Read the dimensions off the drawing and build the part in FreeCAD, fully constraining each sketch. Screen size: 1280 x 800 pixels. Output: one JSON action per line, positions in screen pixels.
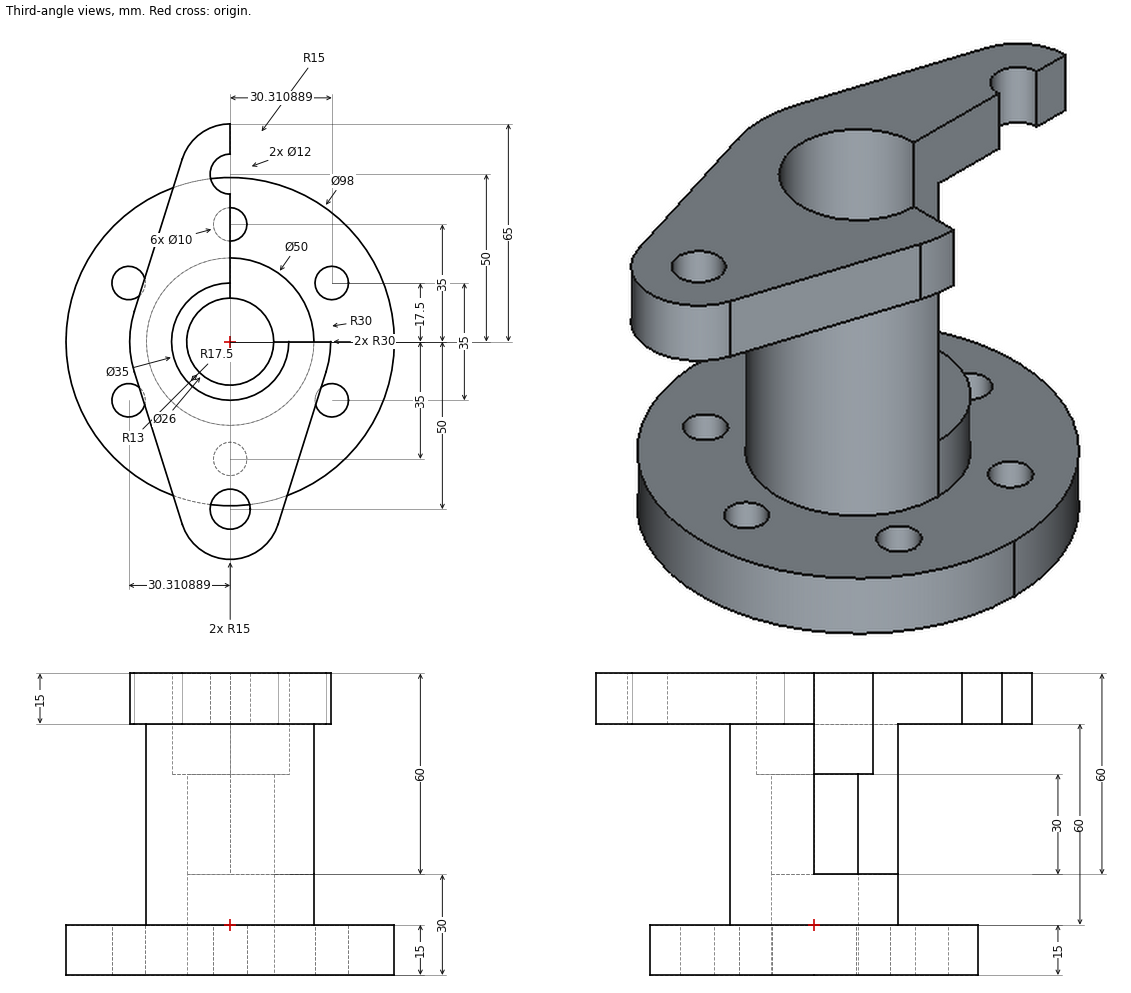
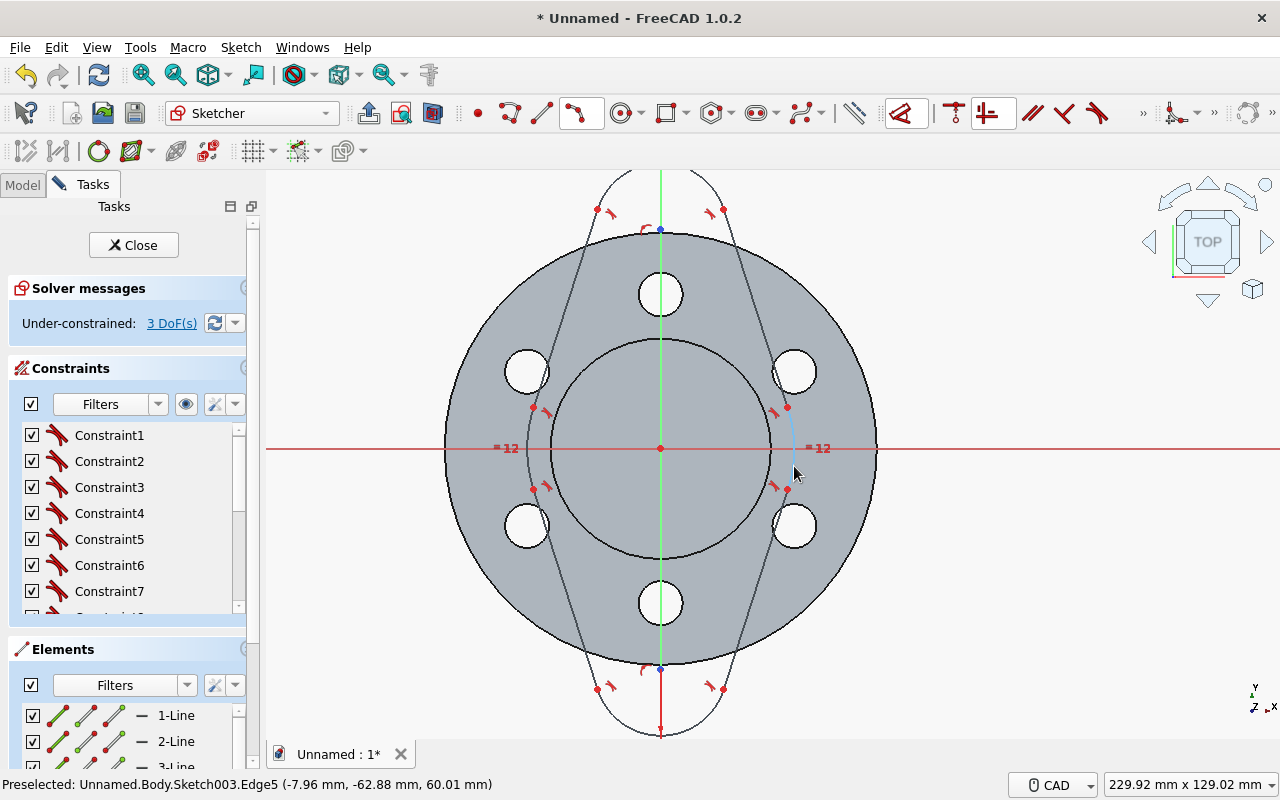
{"action": "left_click", "coordinate": [793, 465]}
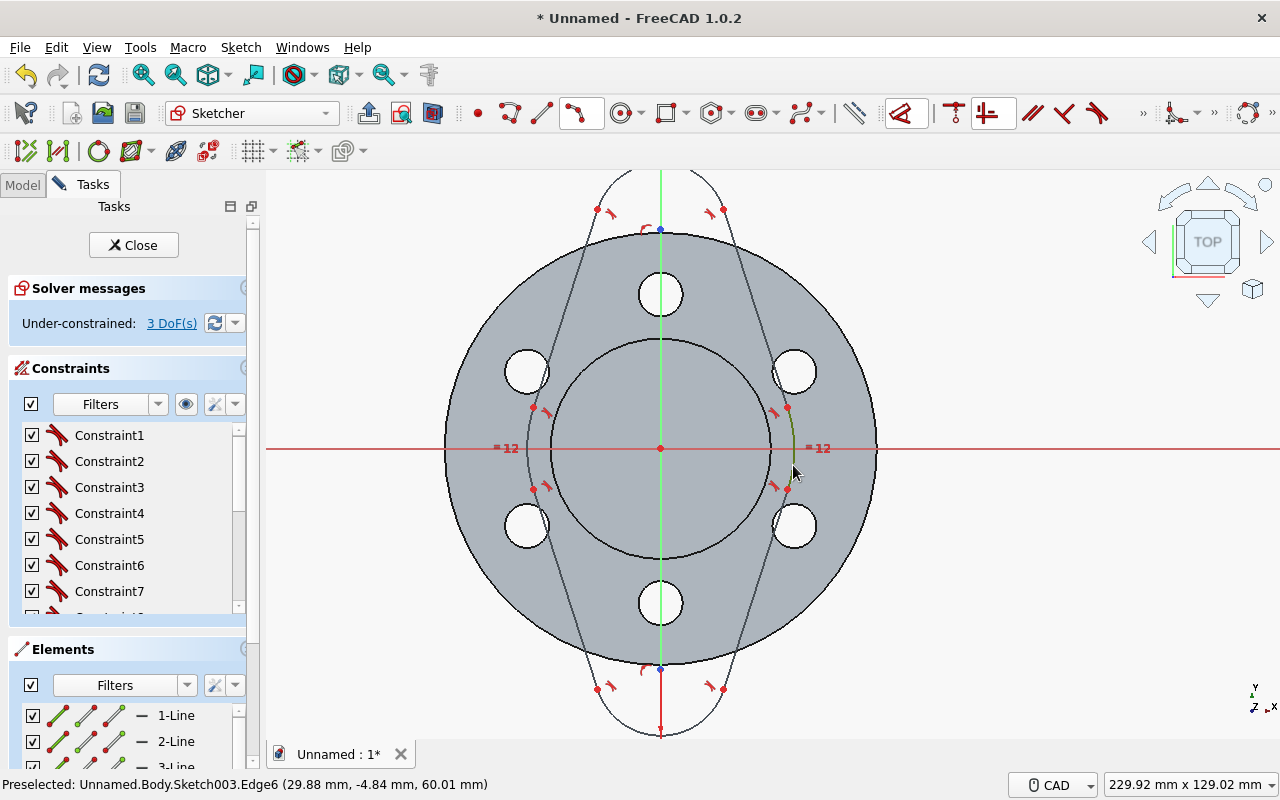
{"action": "key", "text": "k r"}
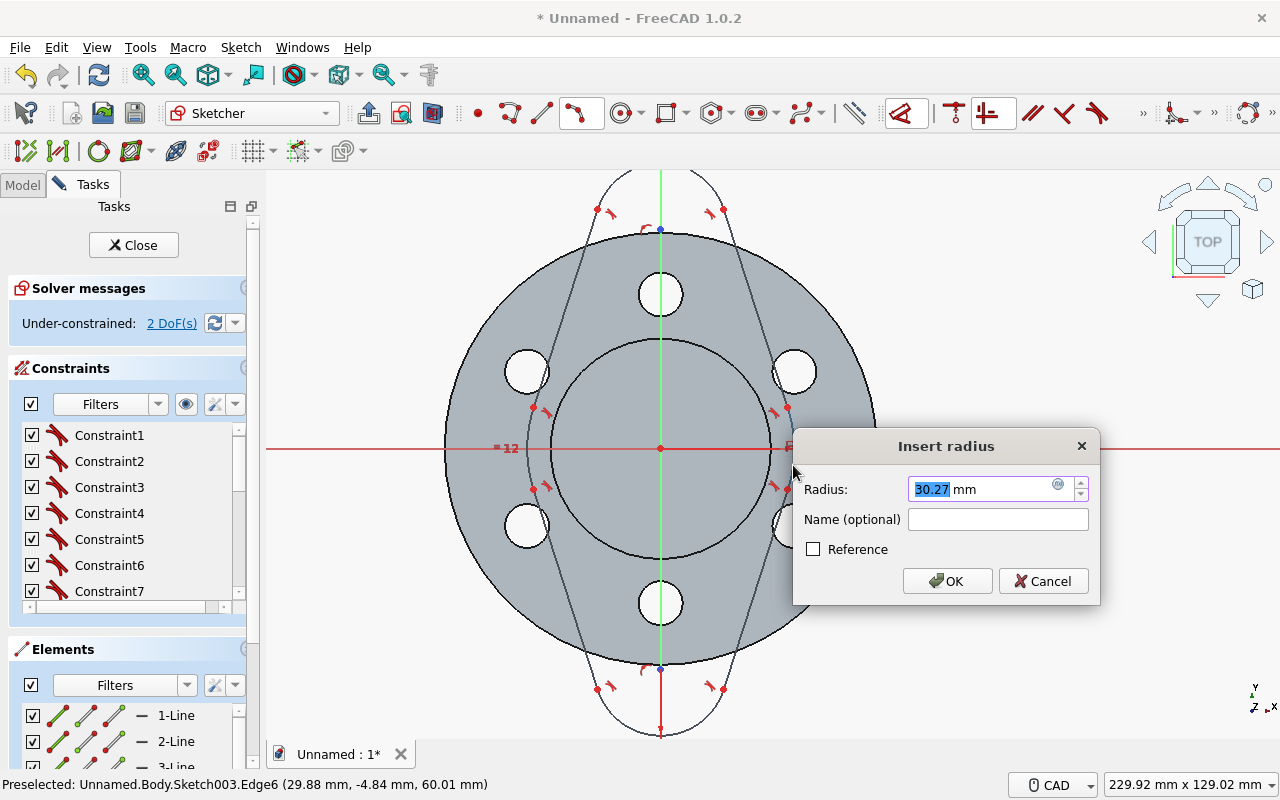
{"action": "type", "text": "30"}
{"action": "key", "text": "Return"}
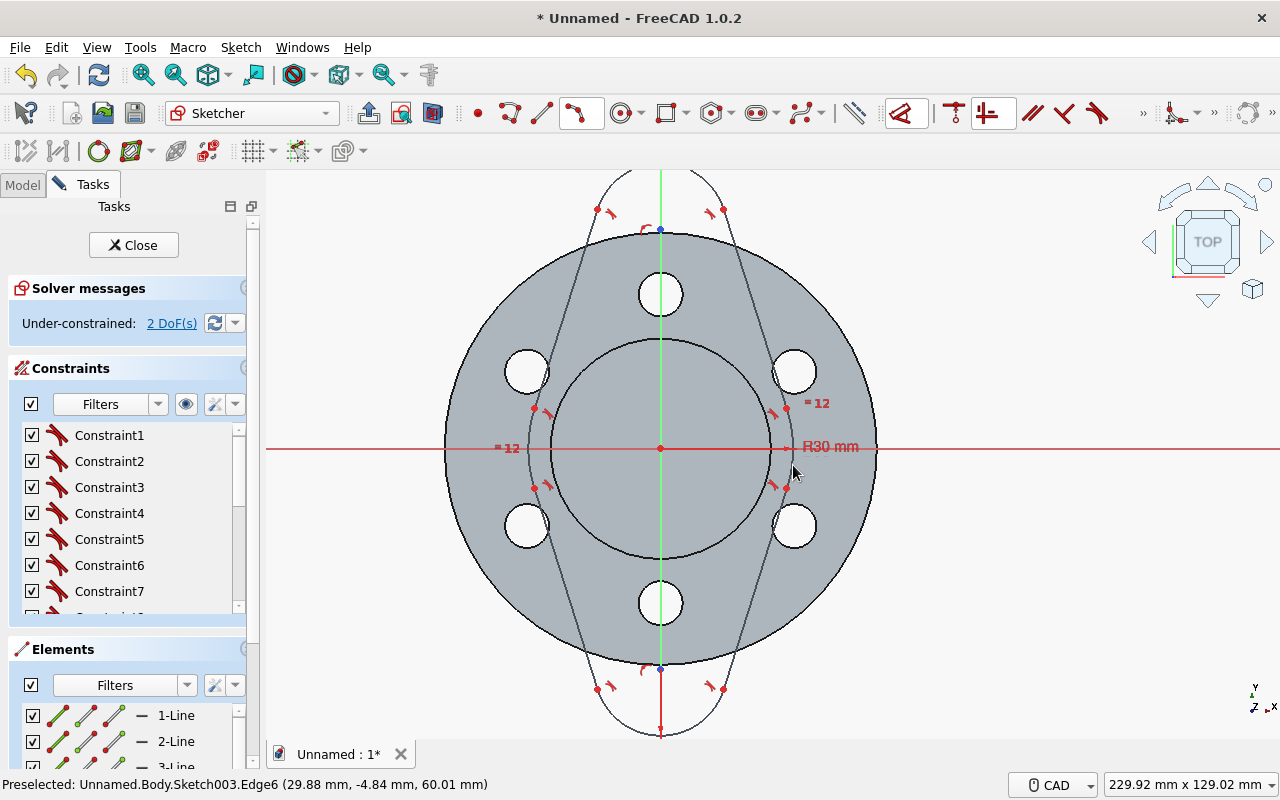
{"action": "left_click", "coordinate": [661, 670]}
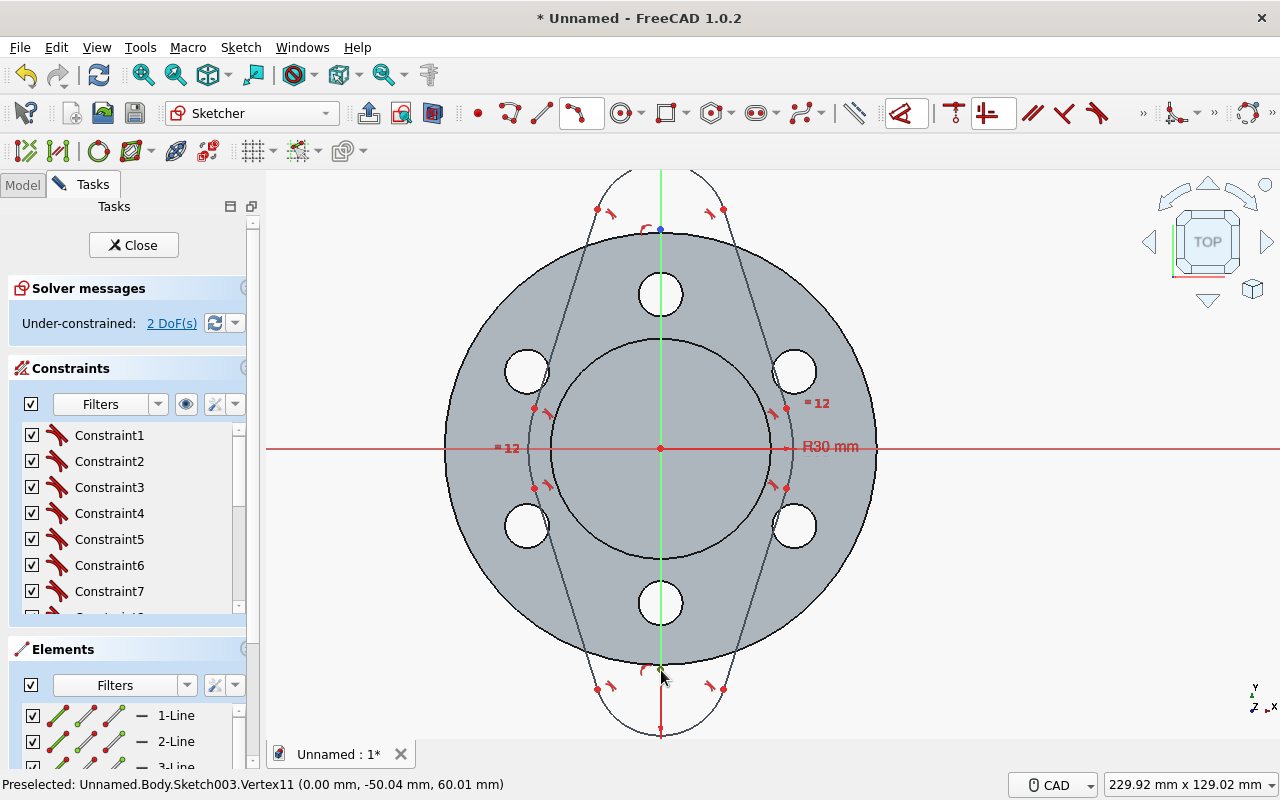
{"action": "key", "text": "i"}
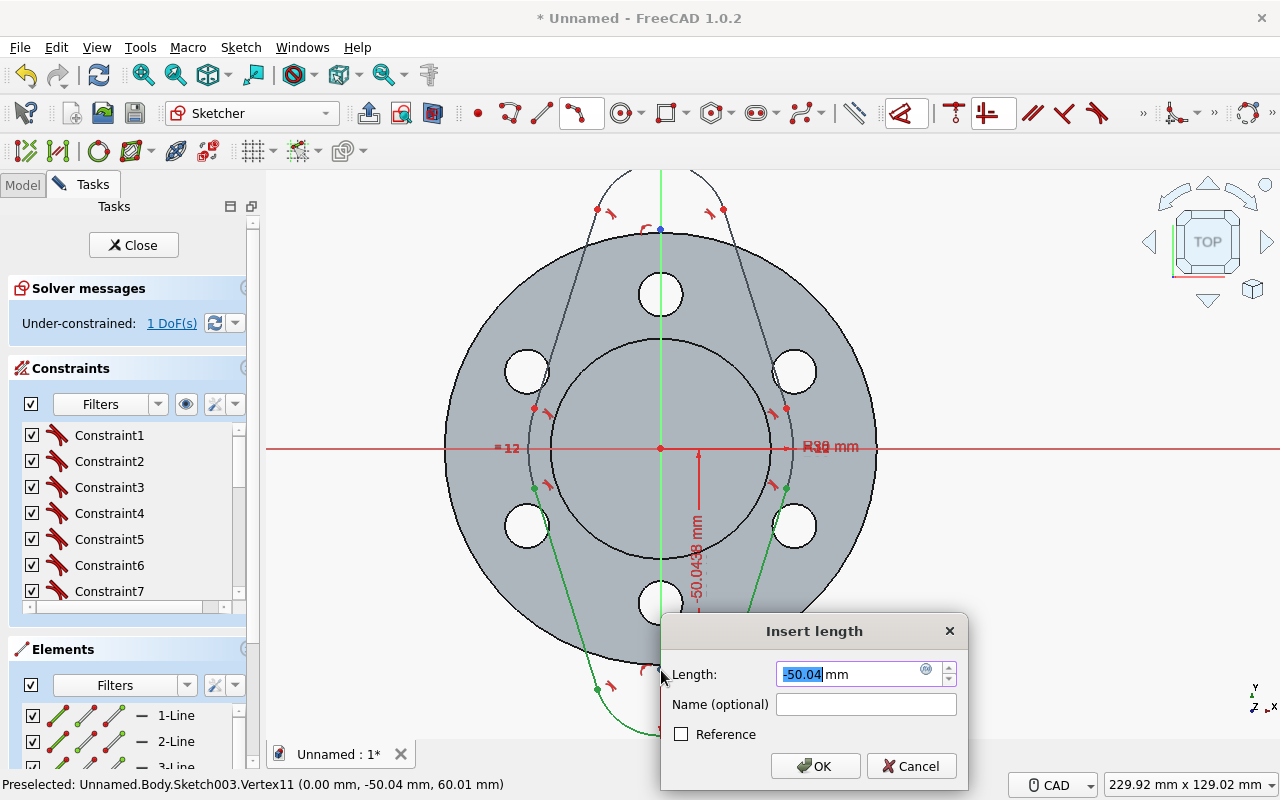
{"action": "type", "text": "-50"}
{"action": "key", "text": "Return"}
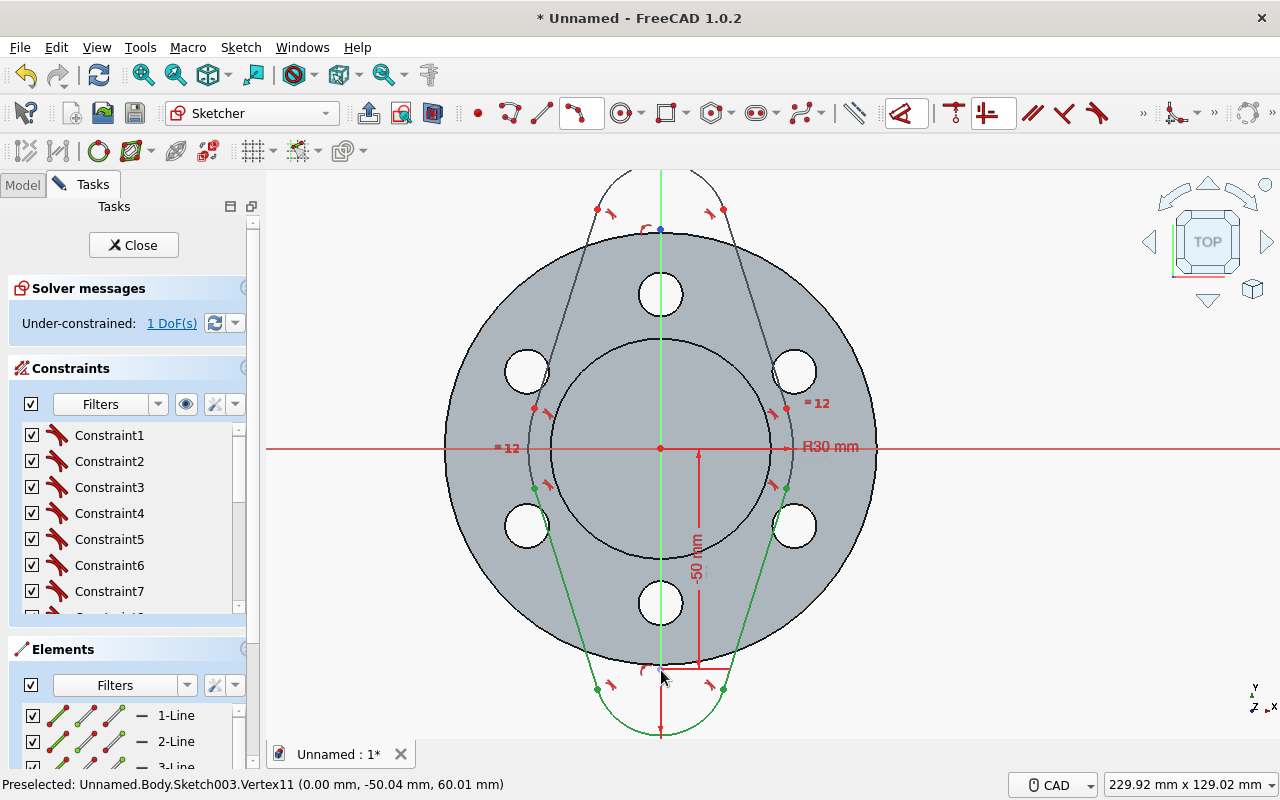
{"action": "left_click", "coordinate": [661, 230]}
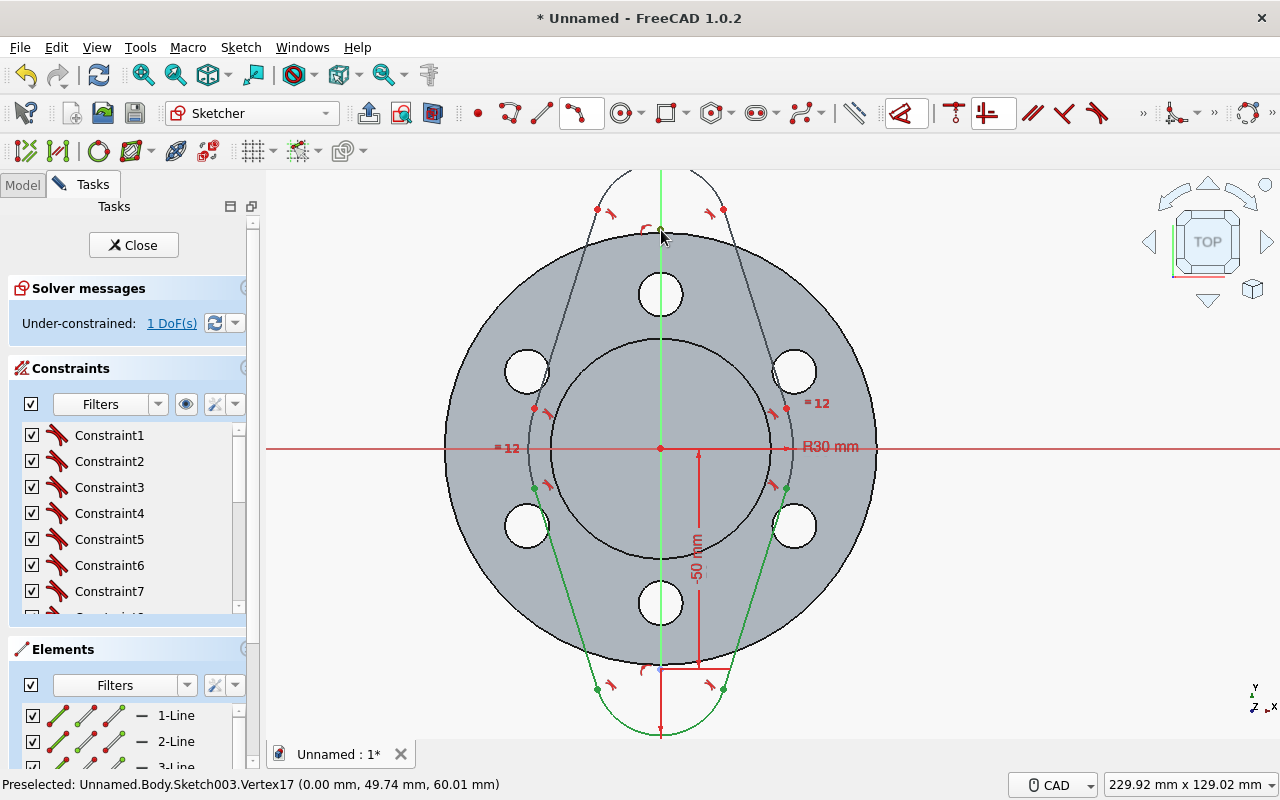
{"action": "key", "text": "i"}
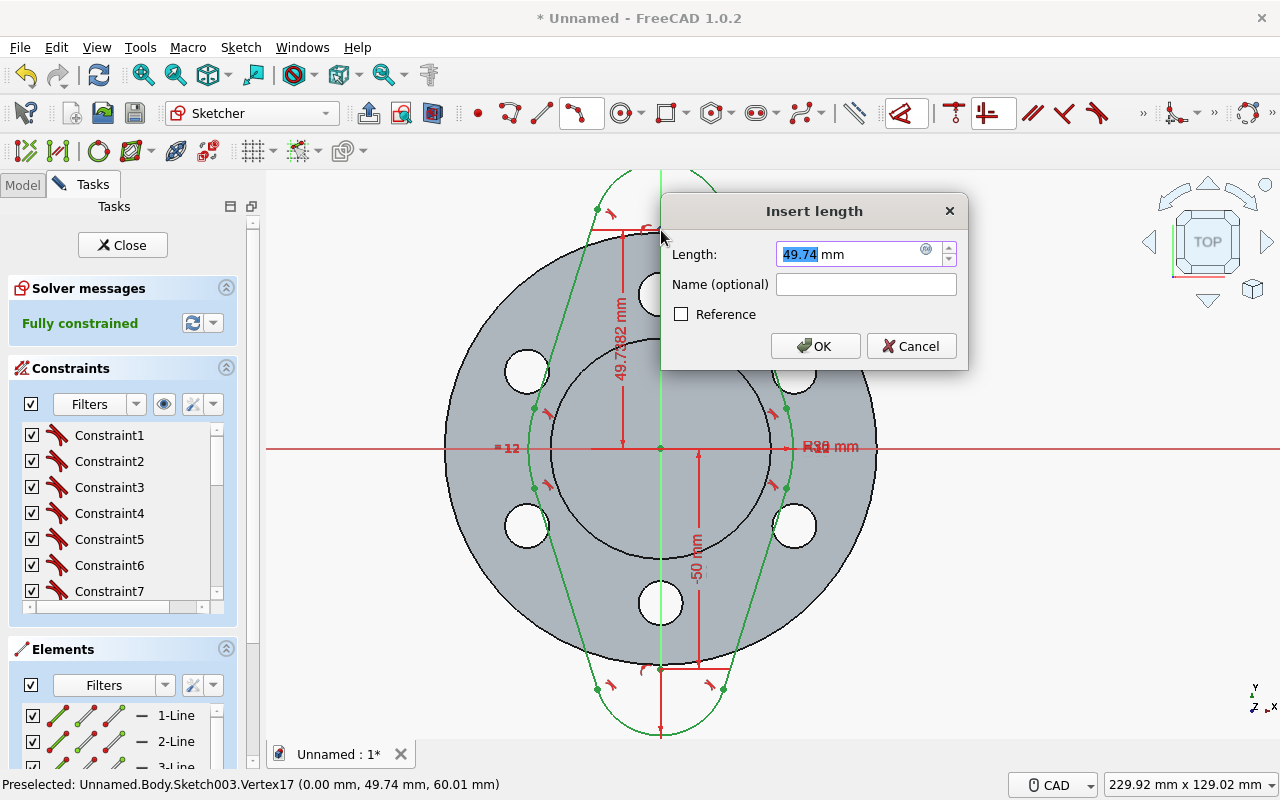
{"action": "type", "text": "50"}
{"action": "key", "text": "Return"}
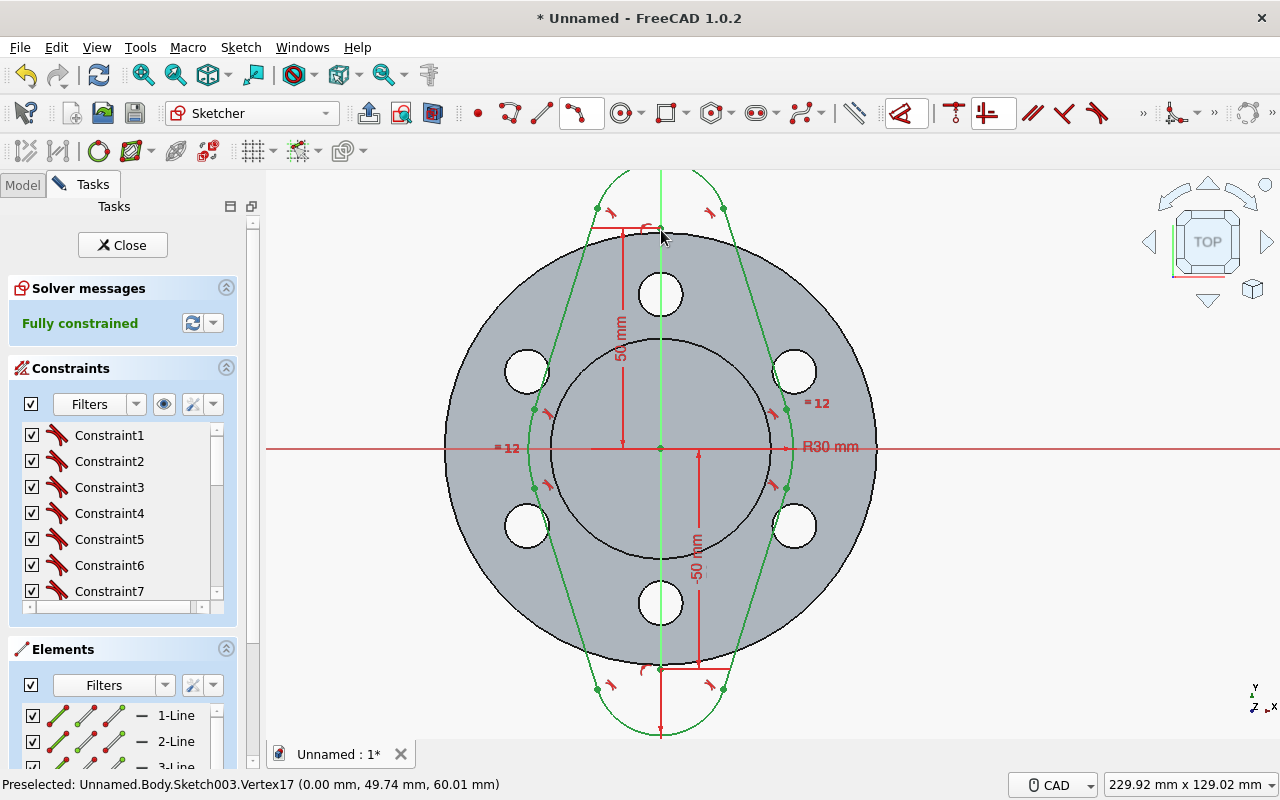
{"action": "left_click", "coordinate": [123, 245]}